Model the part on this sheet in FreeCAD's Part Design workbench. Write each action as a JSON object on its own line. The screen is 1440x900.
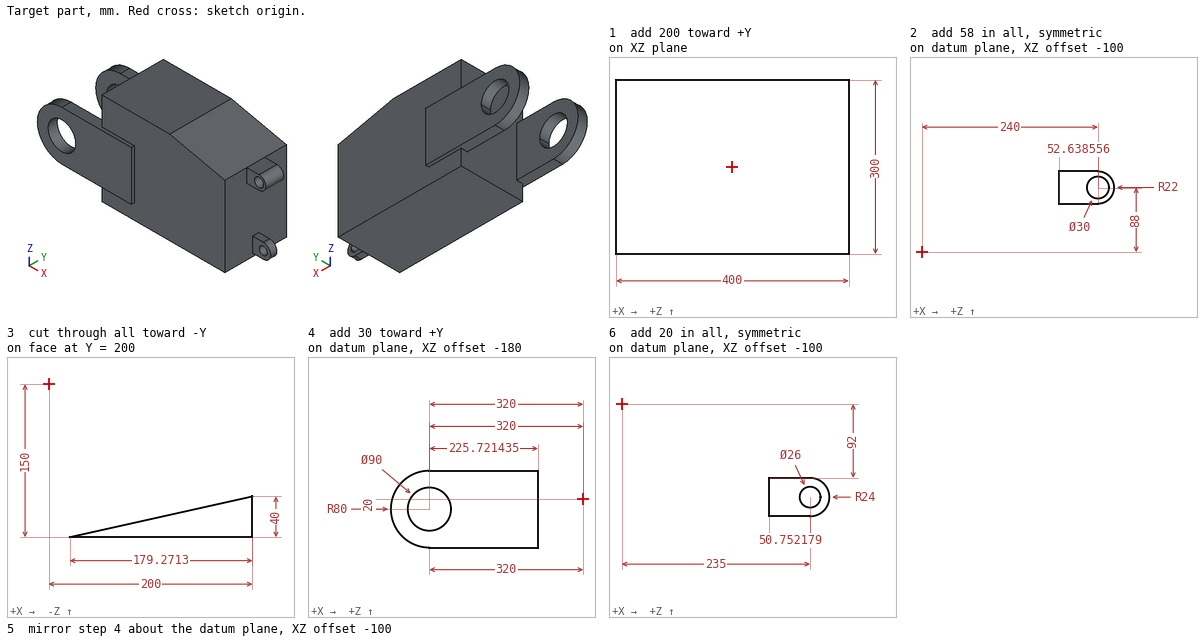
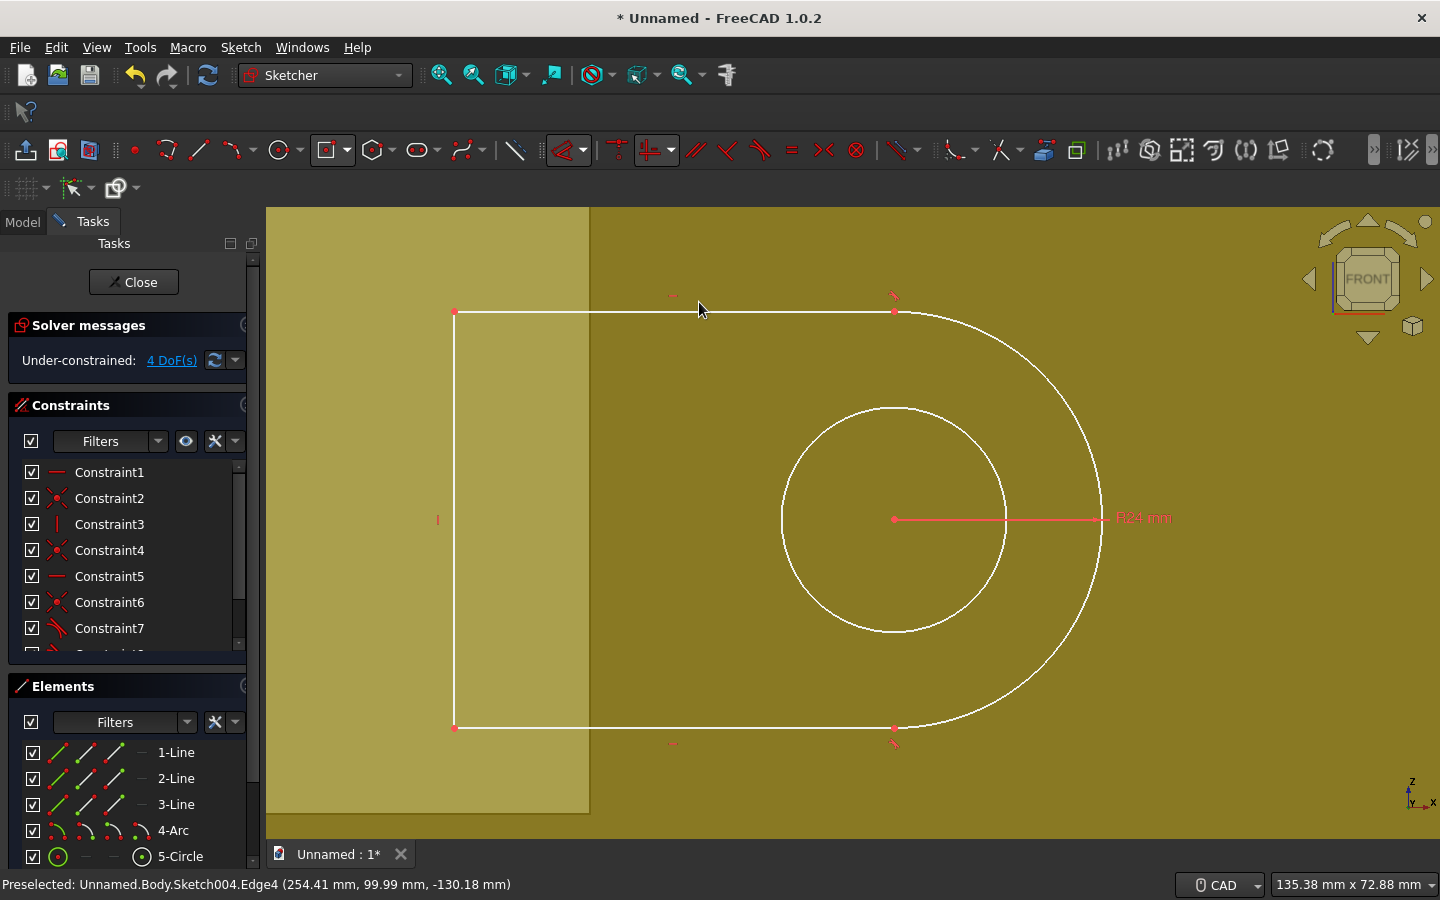
{"action": "left_click", "coordinate": [973, 440]}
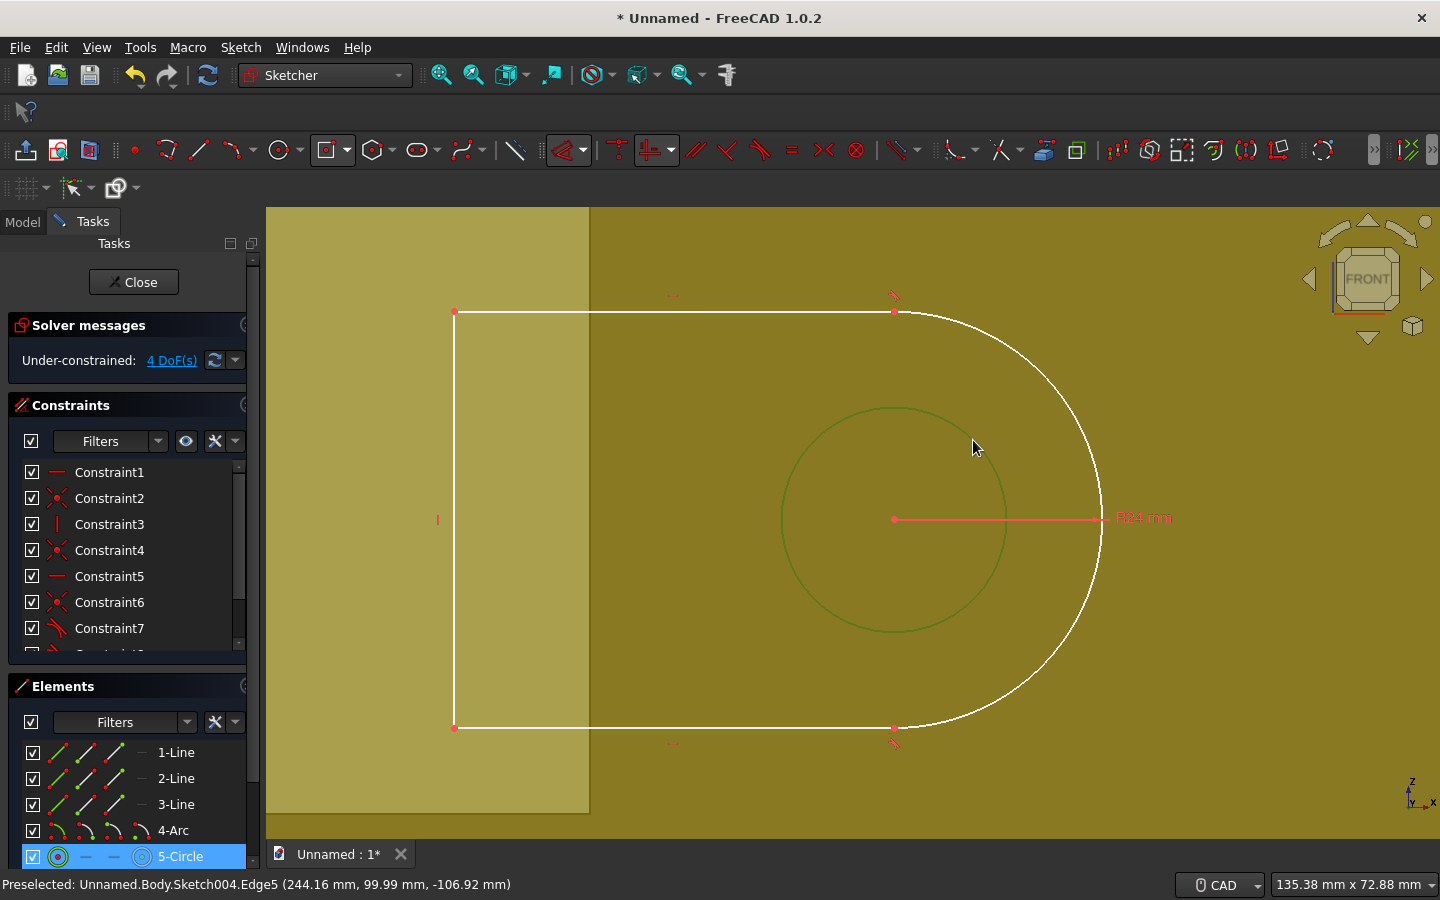
{"action": "key", "text": "k o"}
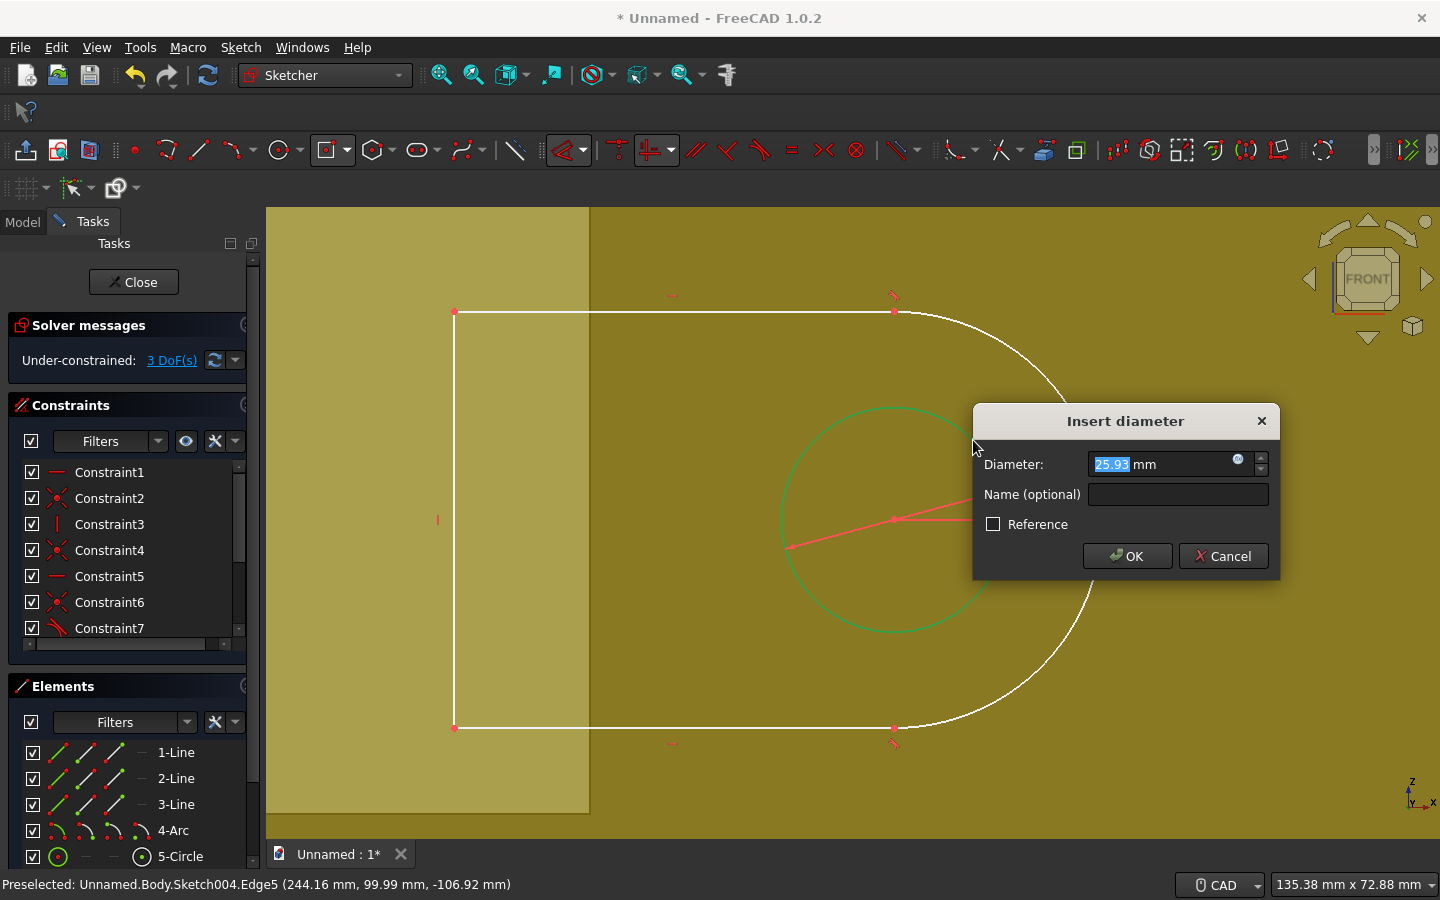
{"action": "type", "text": "26"}
{"action": "key", "text": "Return"}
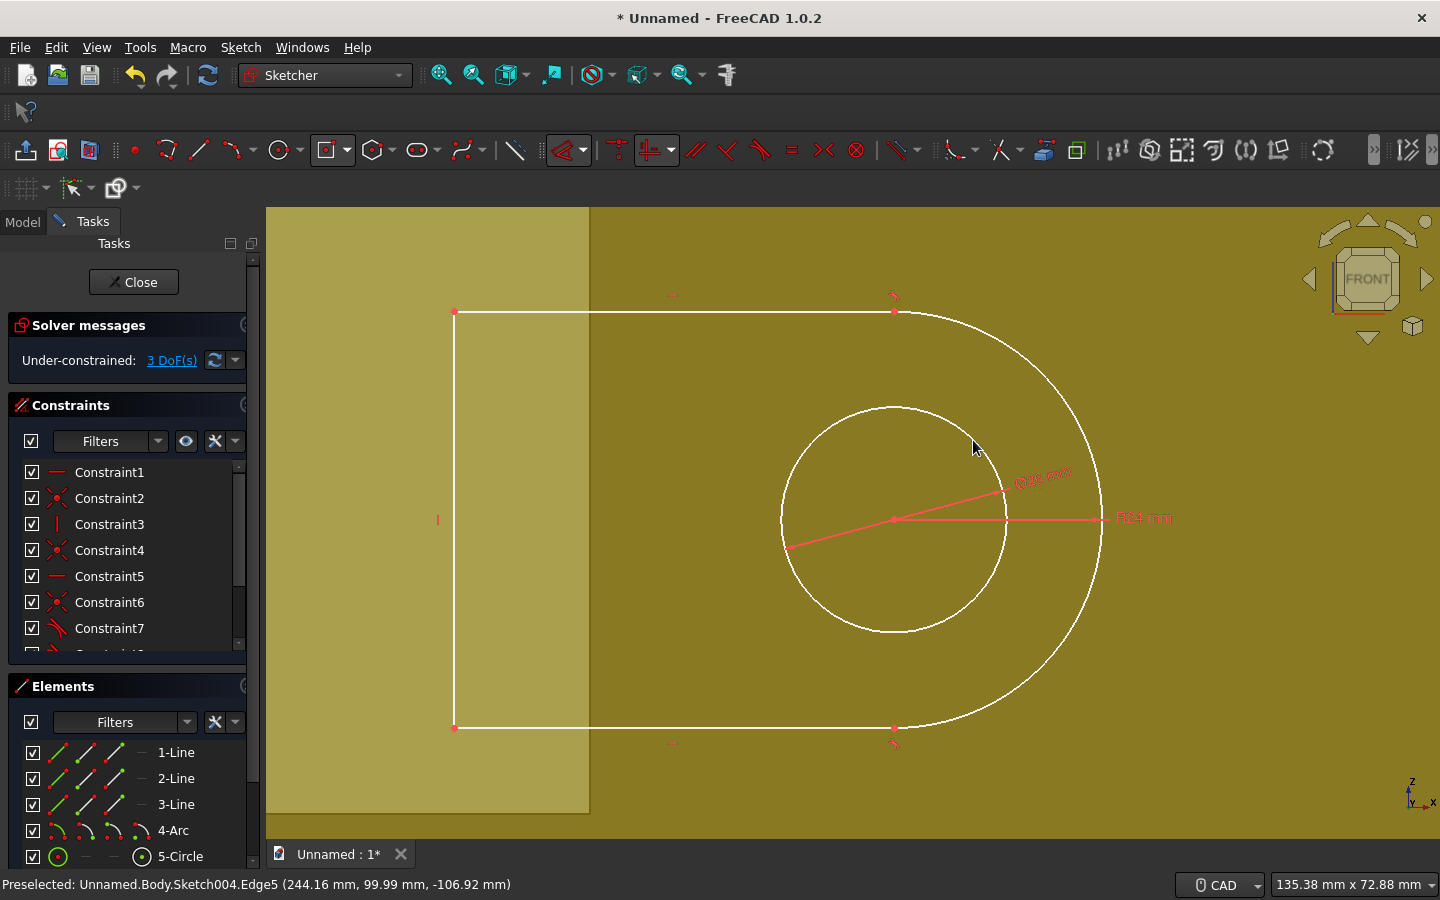
{"action": "left_click", "coordinate": [454, 312]}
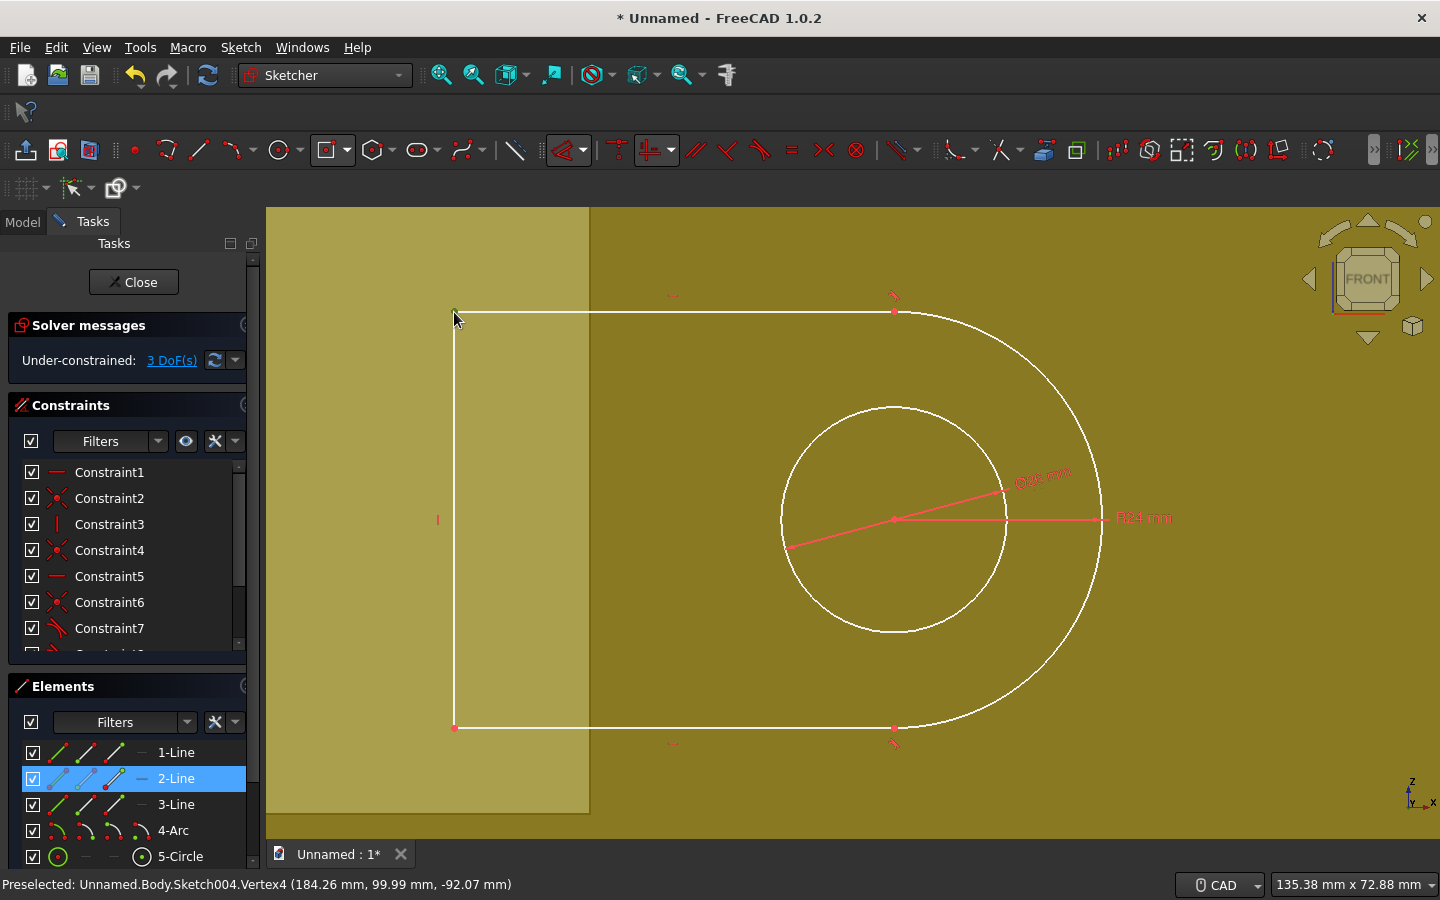
{"action": "key", "text": "i"}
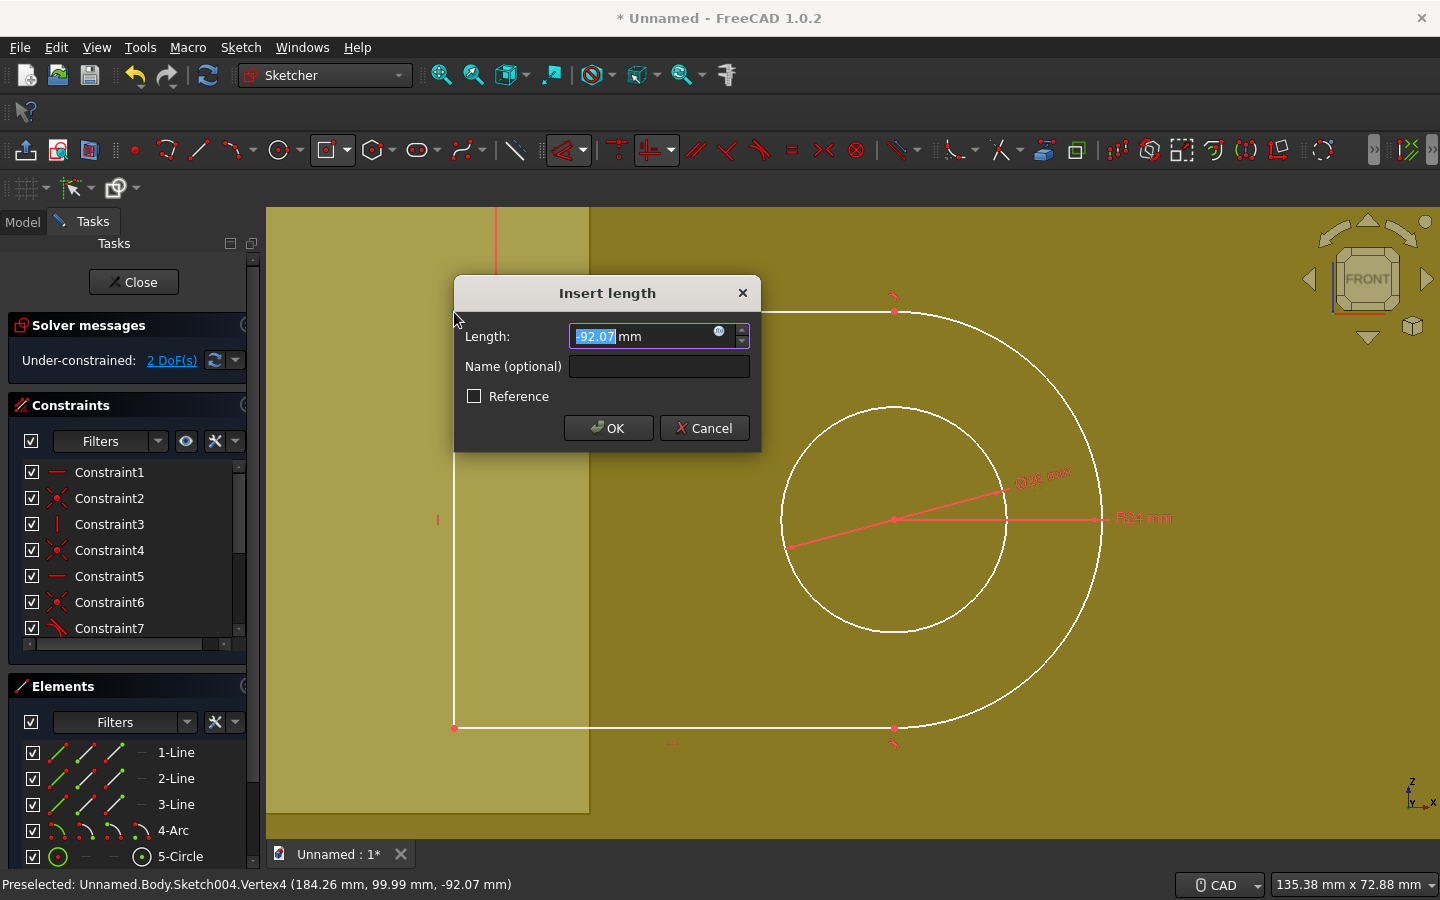
{"action": "type", "text": "-92"}
{"action": "key", "text": "Return"}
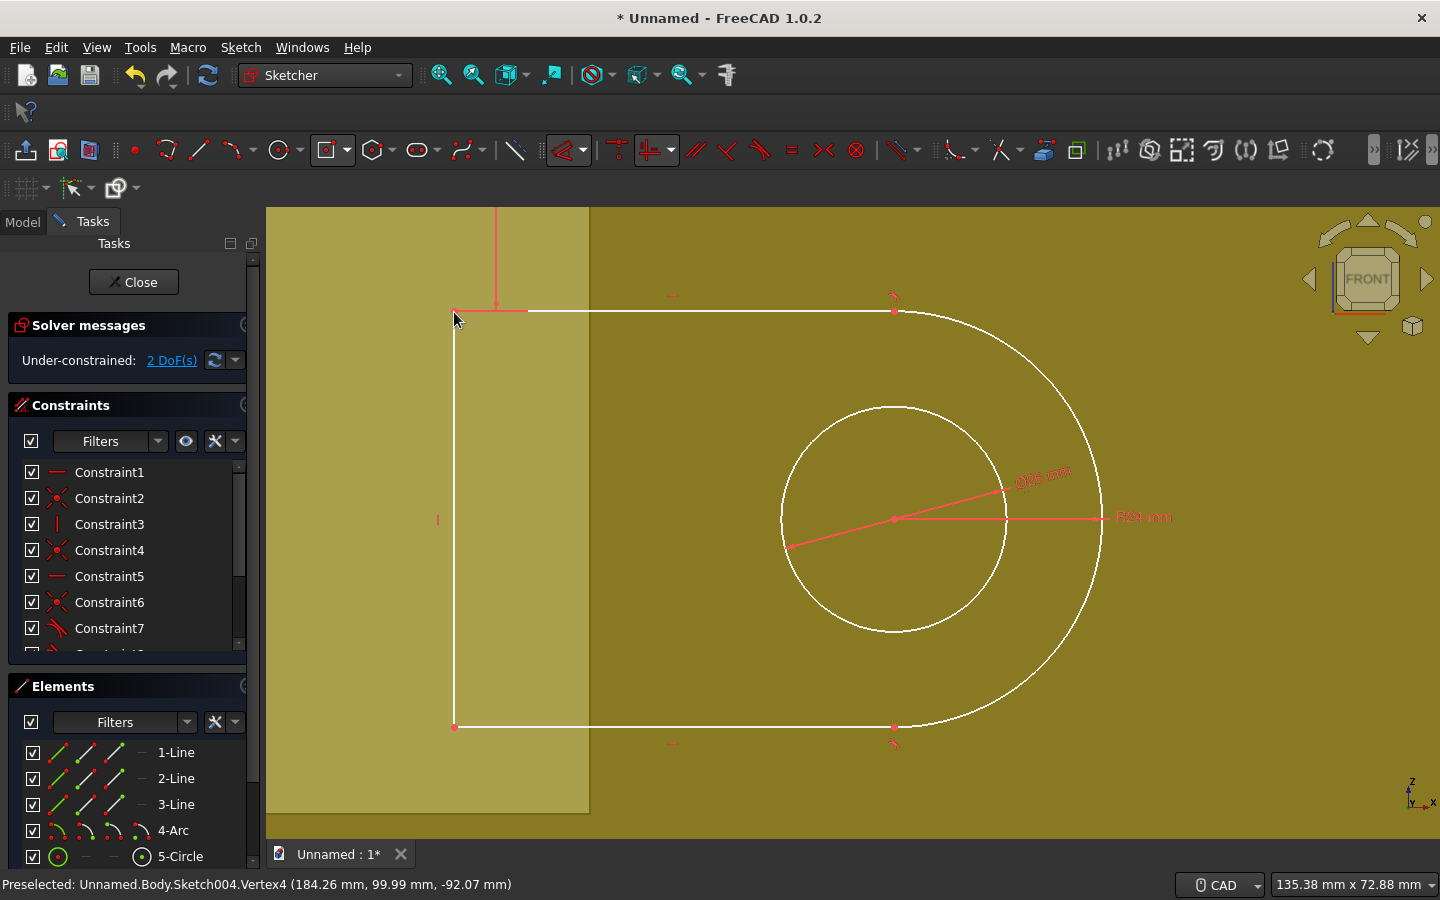
{"action": "left_click", "coordinate": [894, 519]}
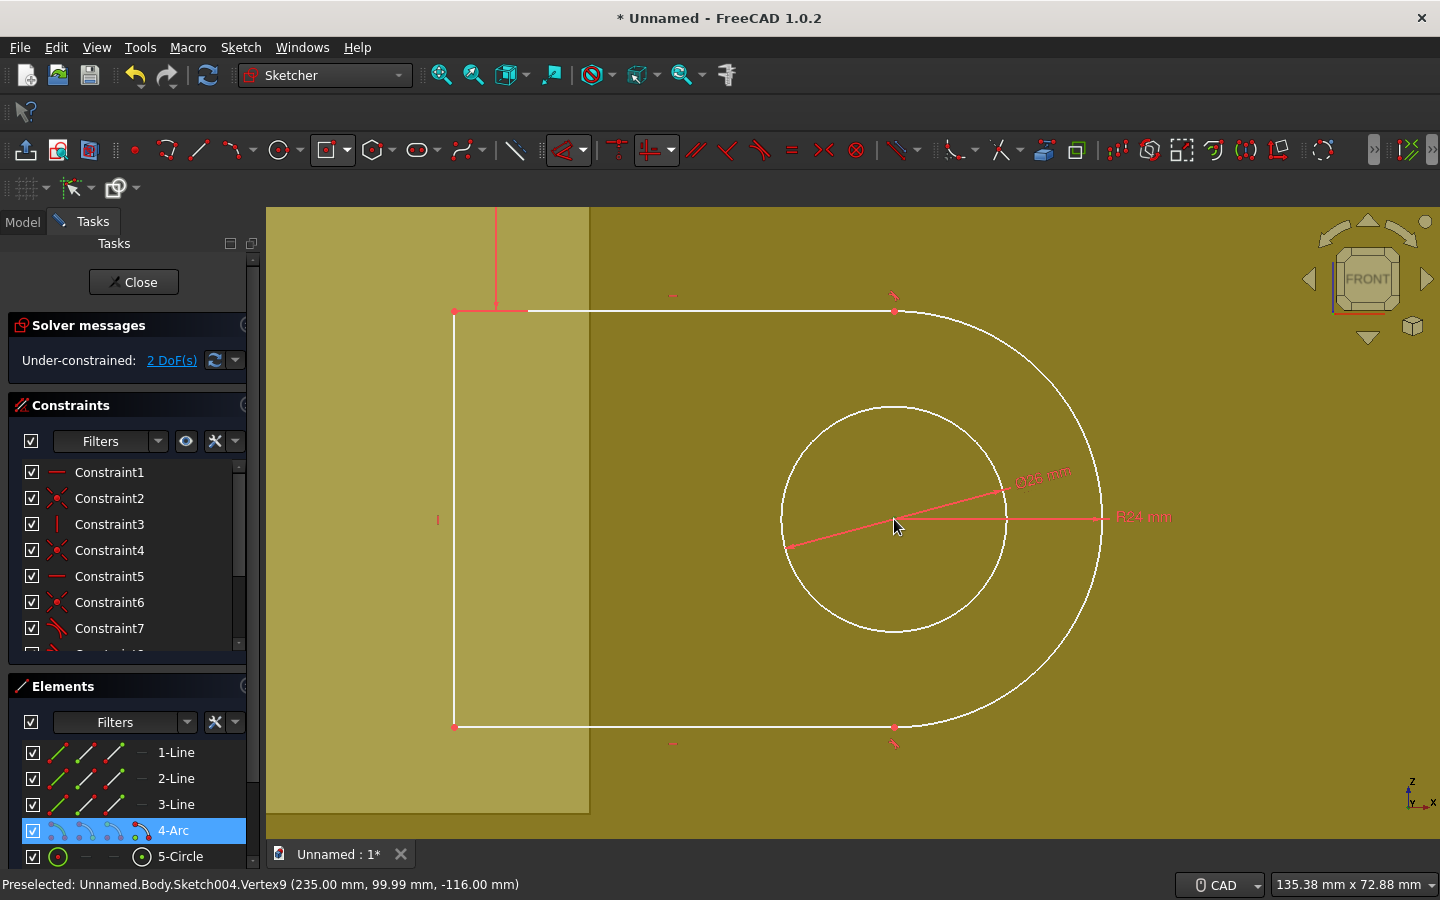
{"action": "left_click", "coordinate": [586, 150]}